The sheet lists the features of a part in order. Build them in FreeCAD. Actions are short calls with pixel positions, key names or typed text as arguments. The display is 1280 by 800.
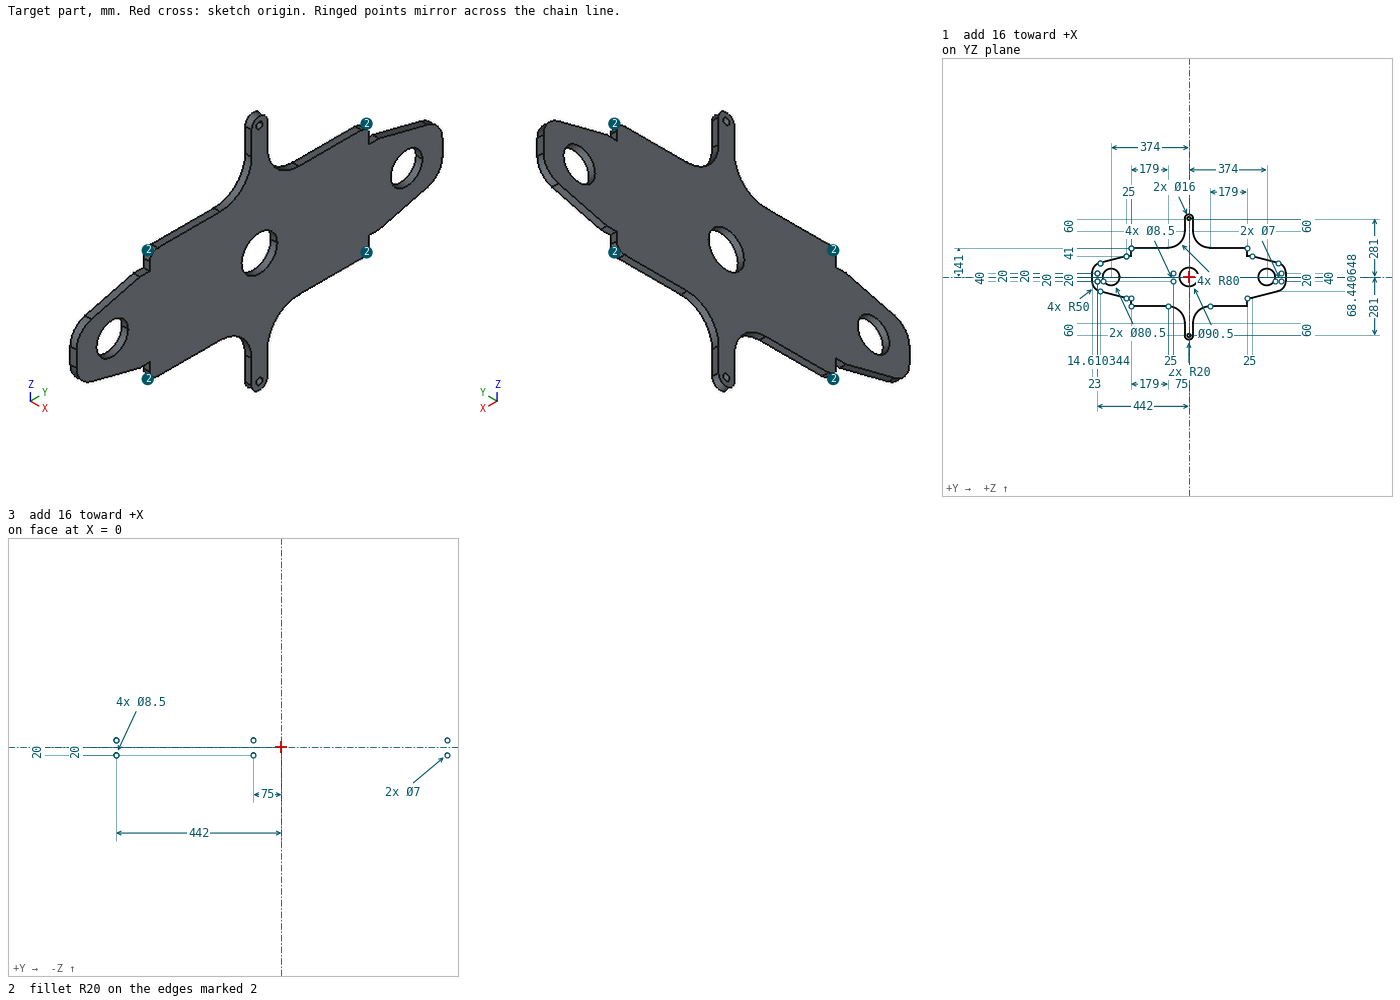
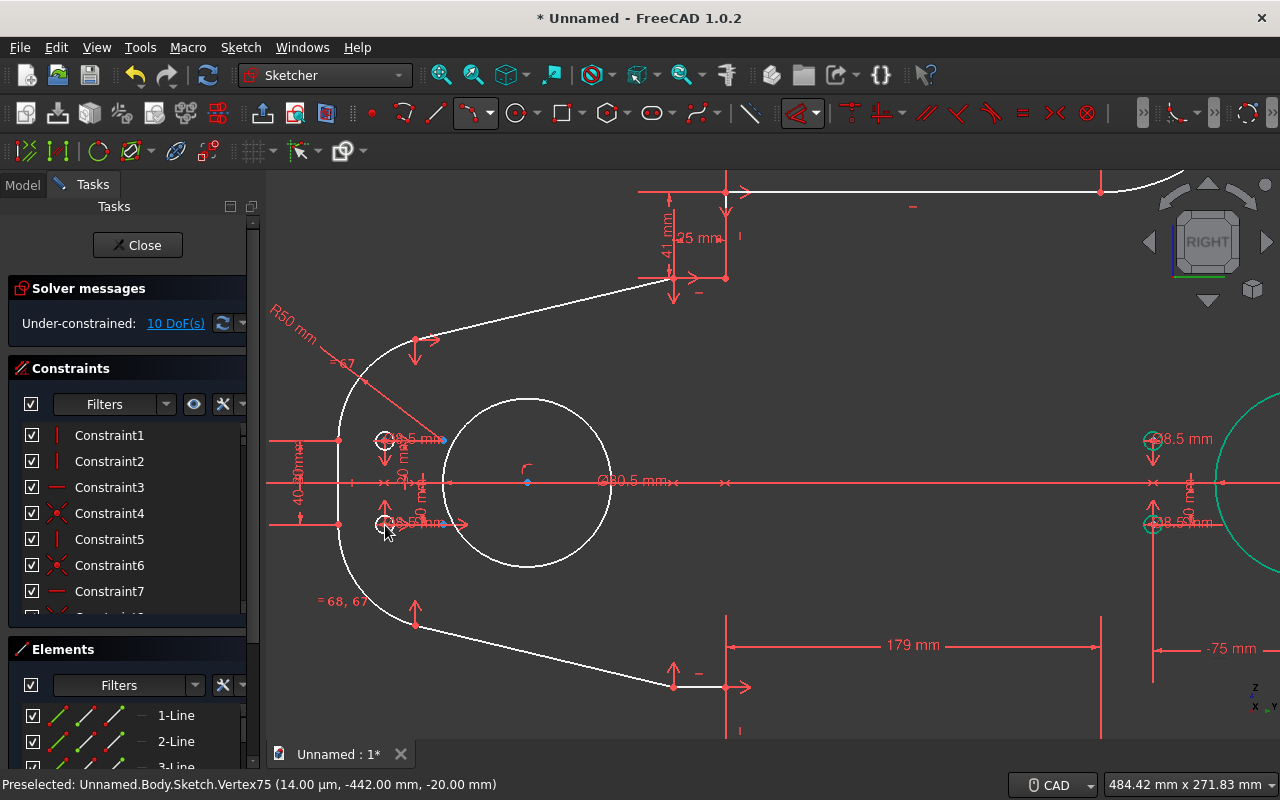
key(l)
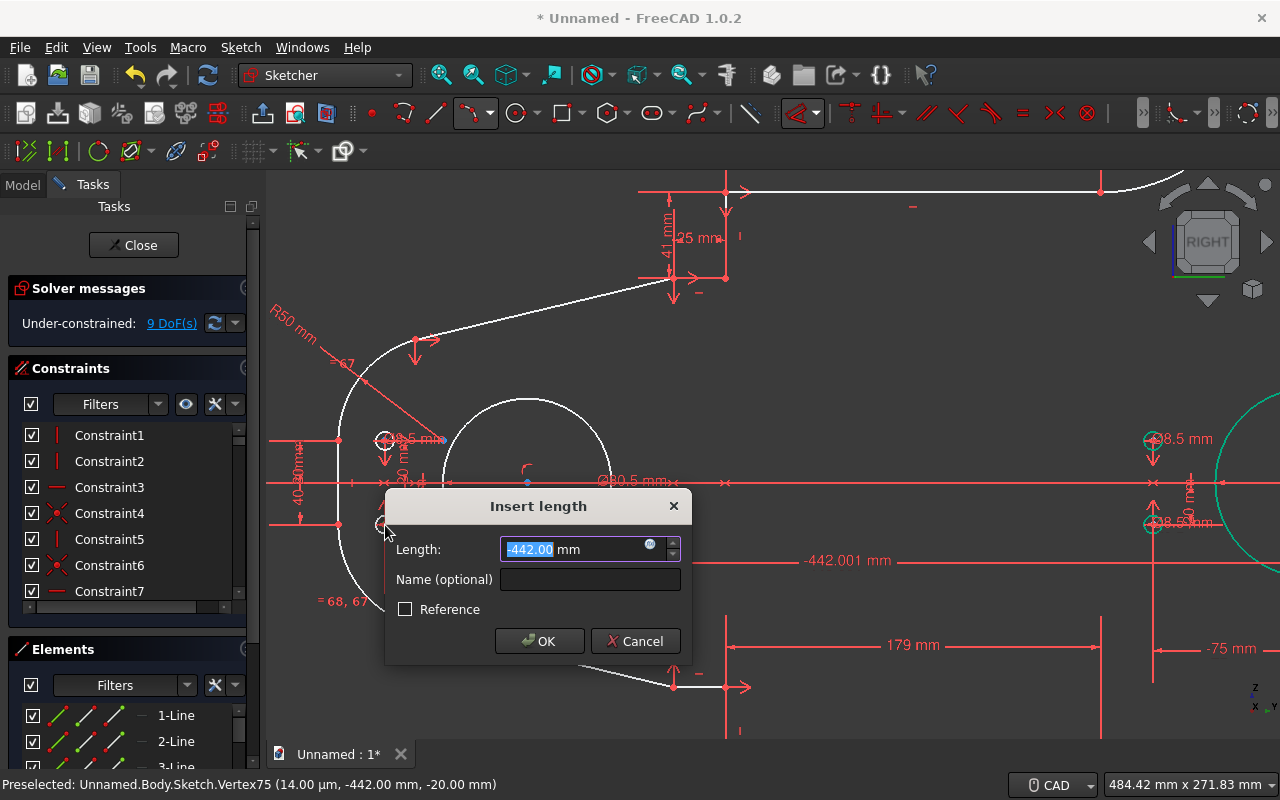
text(-442)
key(Return)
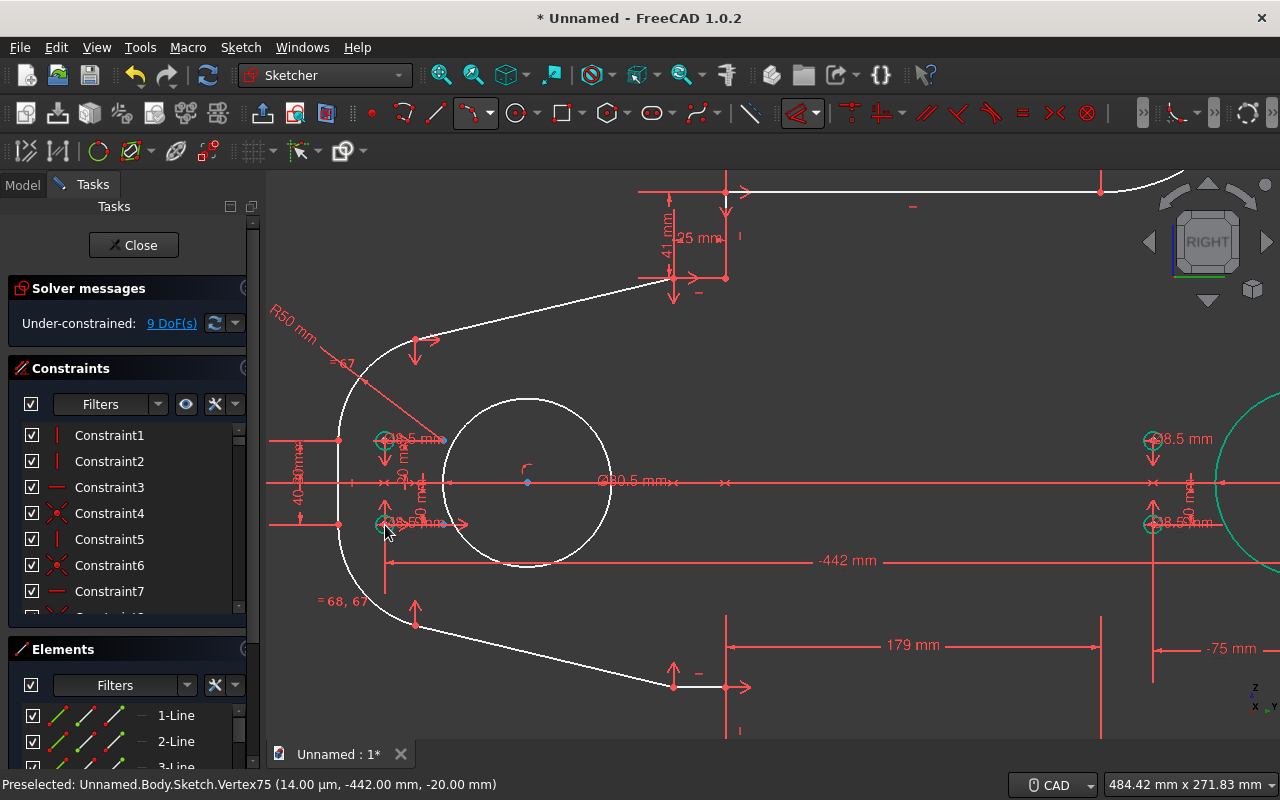
click(527, 483)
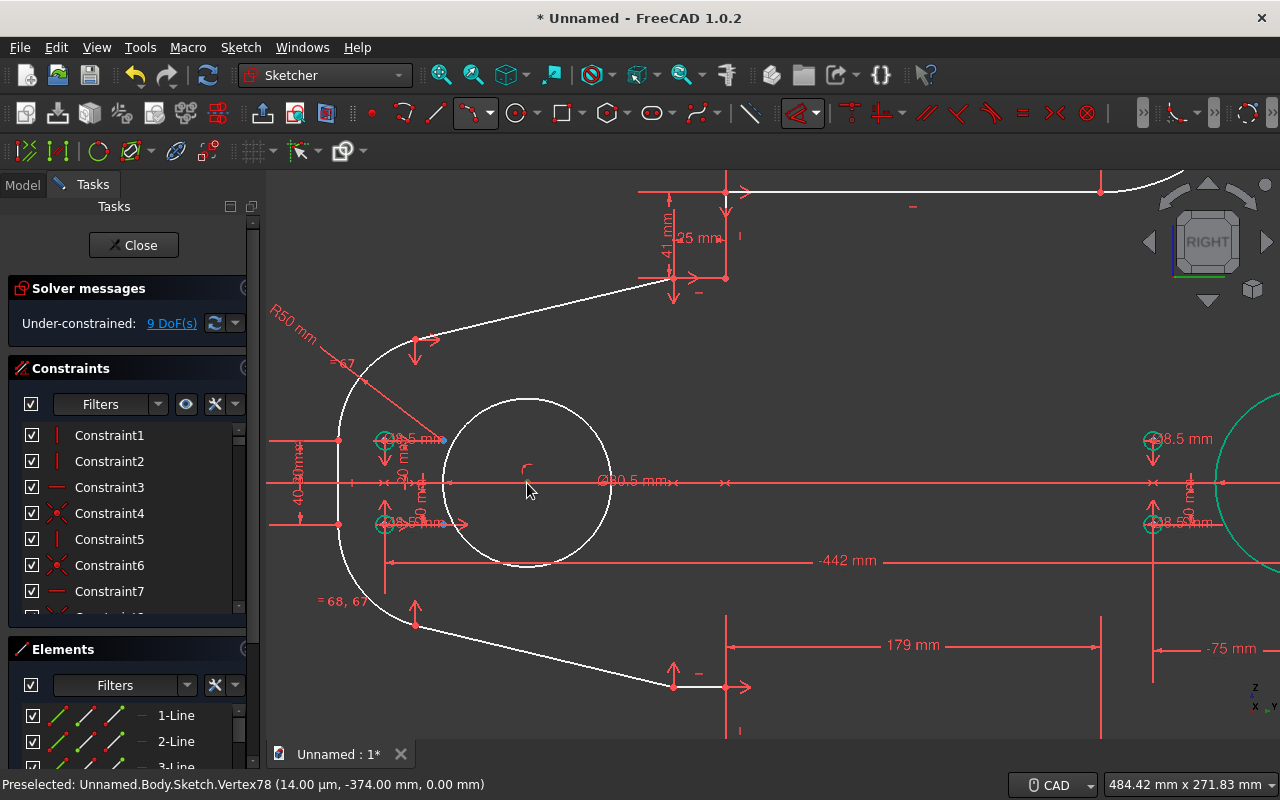
key(l)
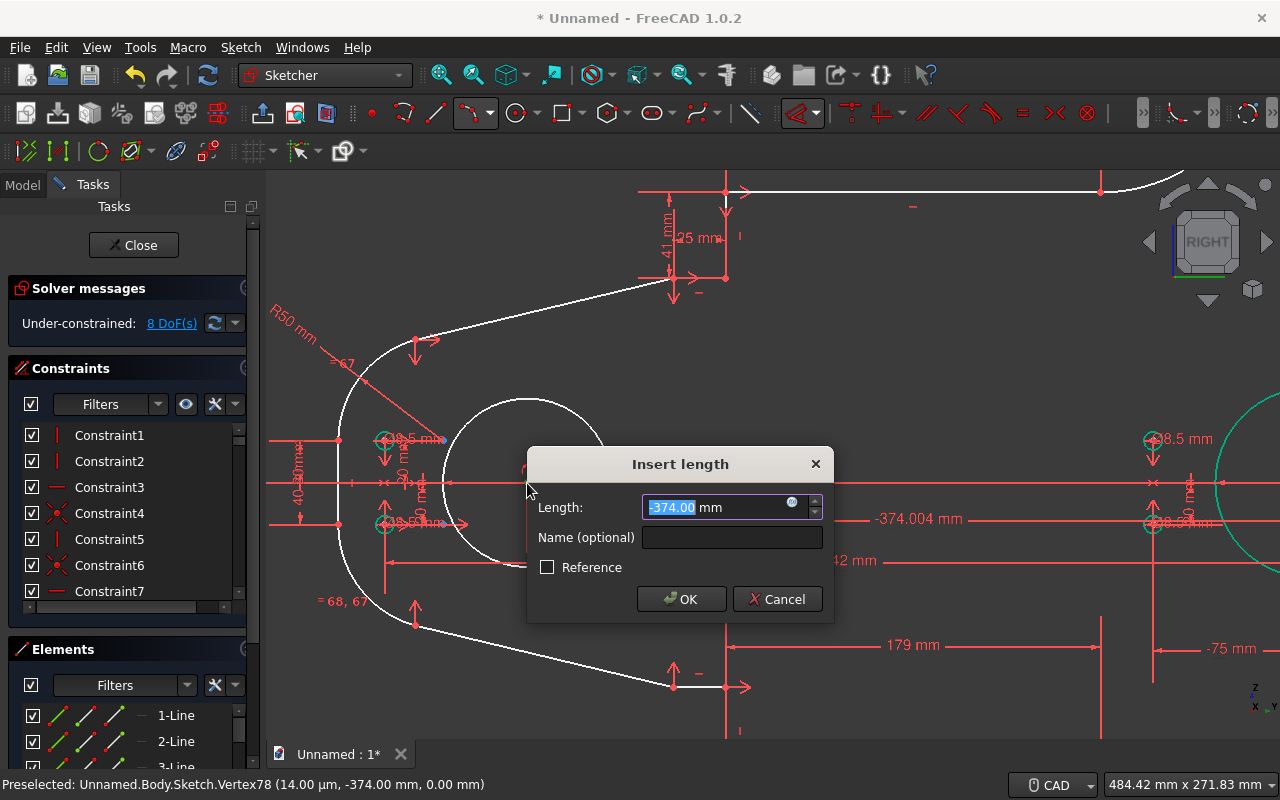
text(-374)
key(Return)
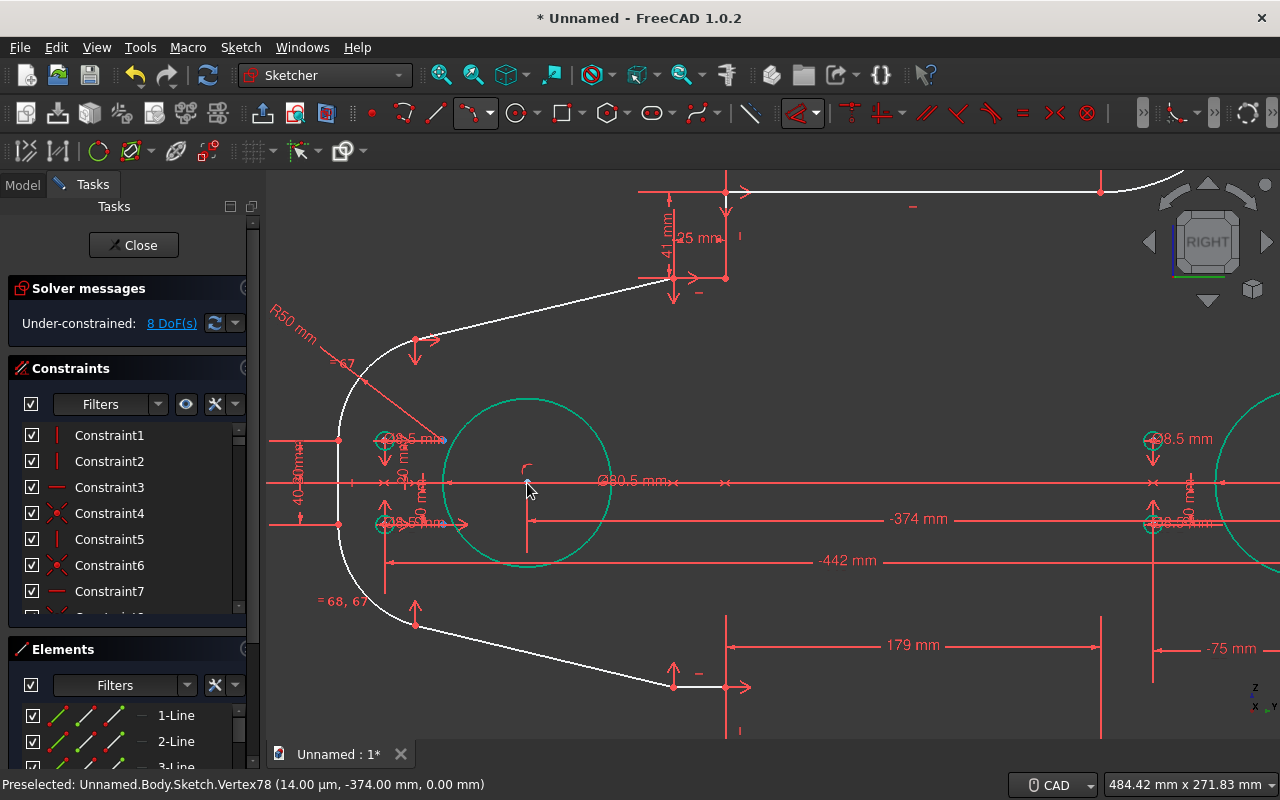
scroll(443, 442, down, 6)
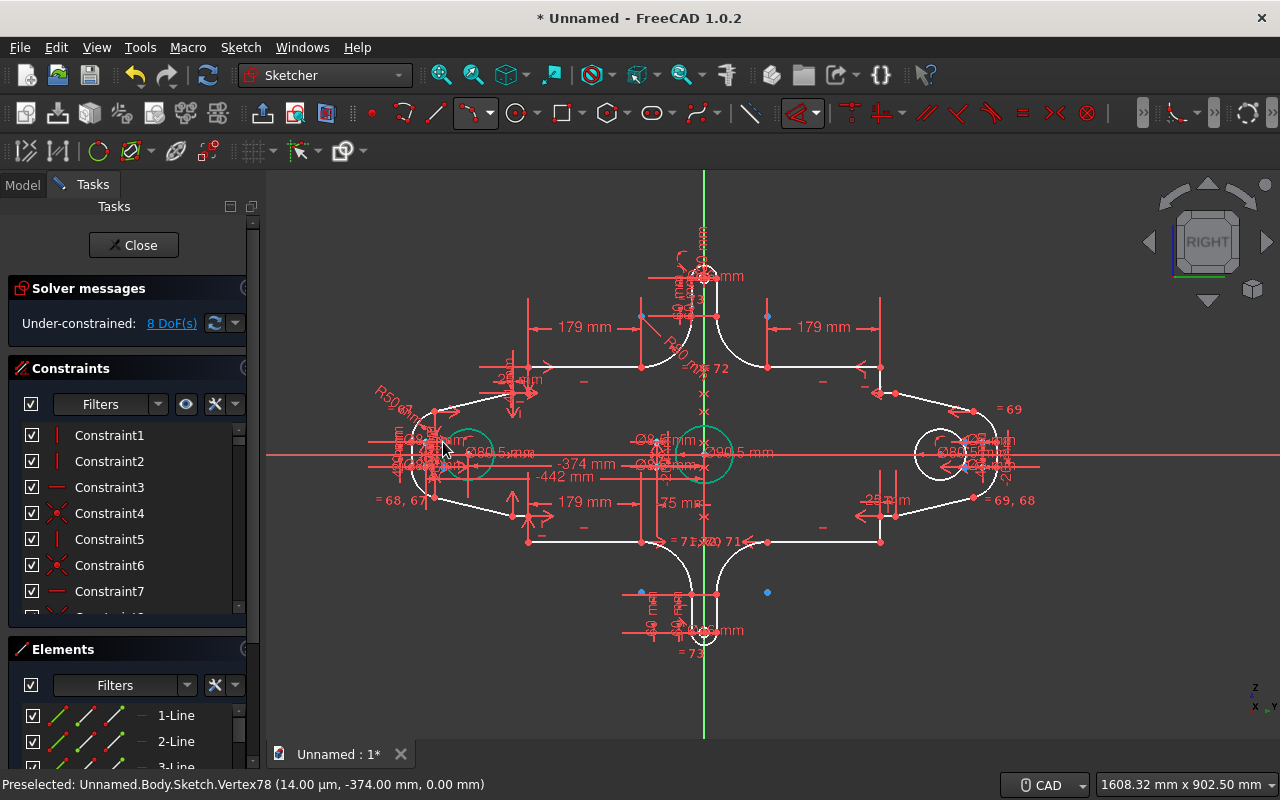
click(704, 633)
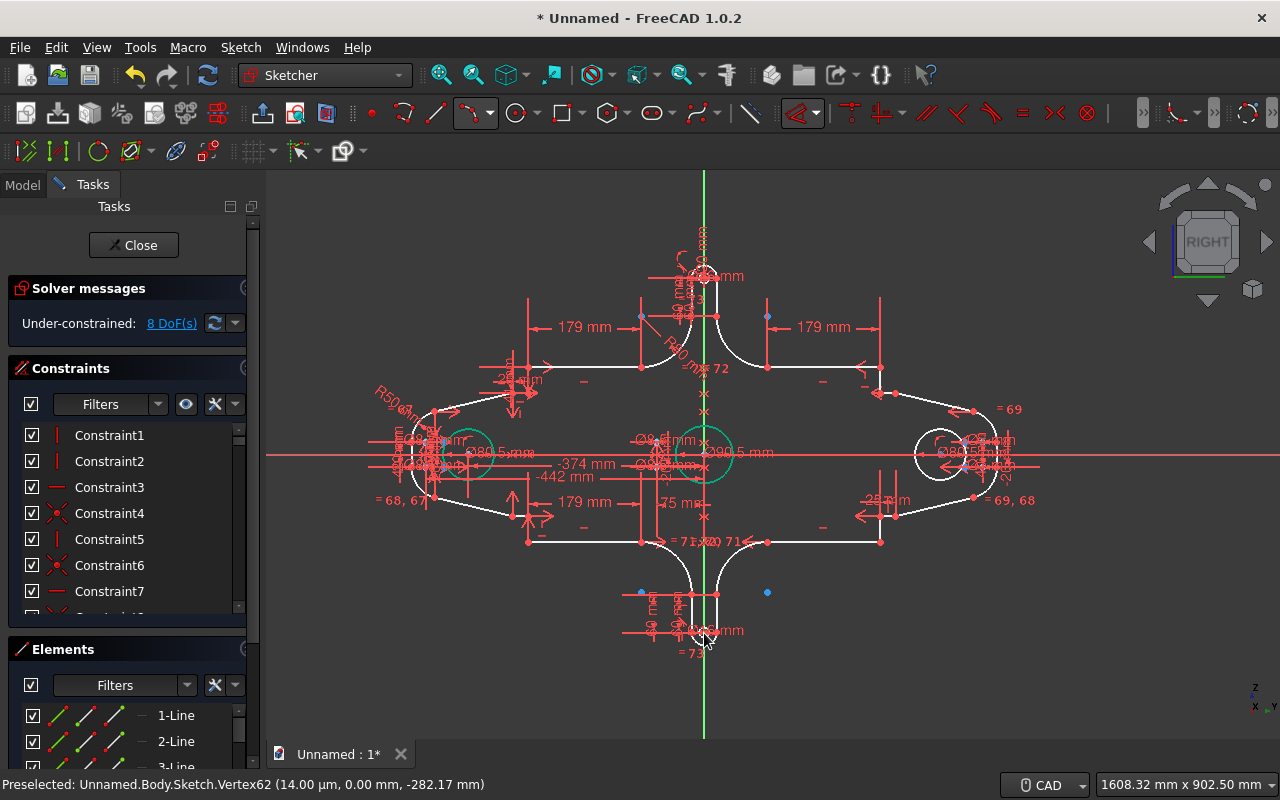
key(i)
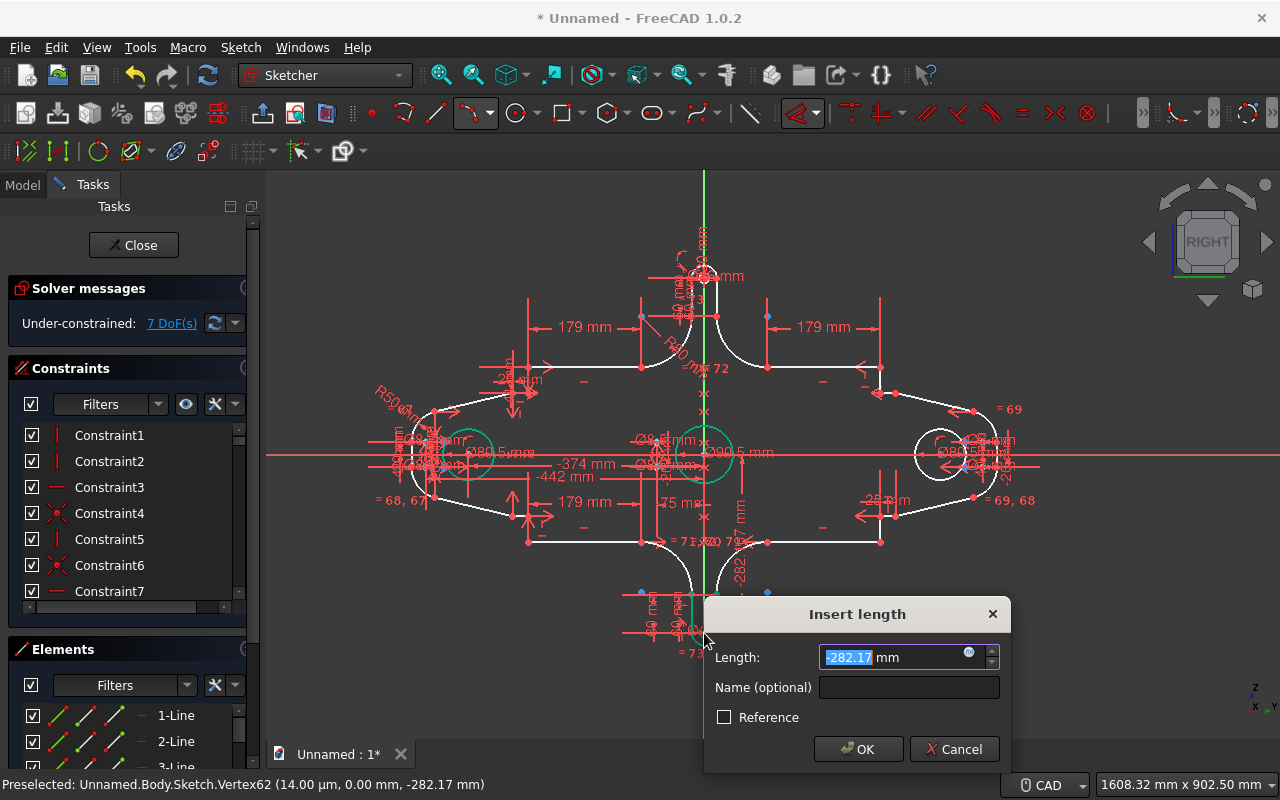
text(-281)
key(Return)